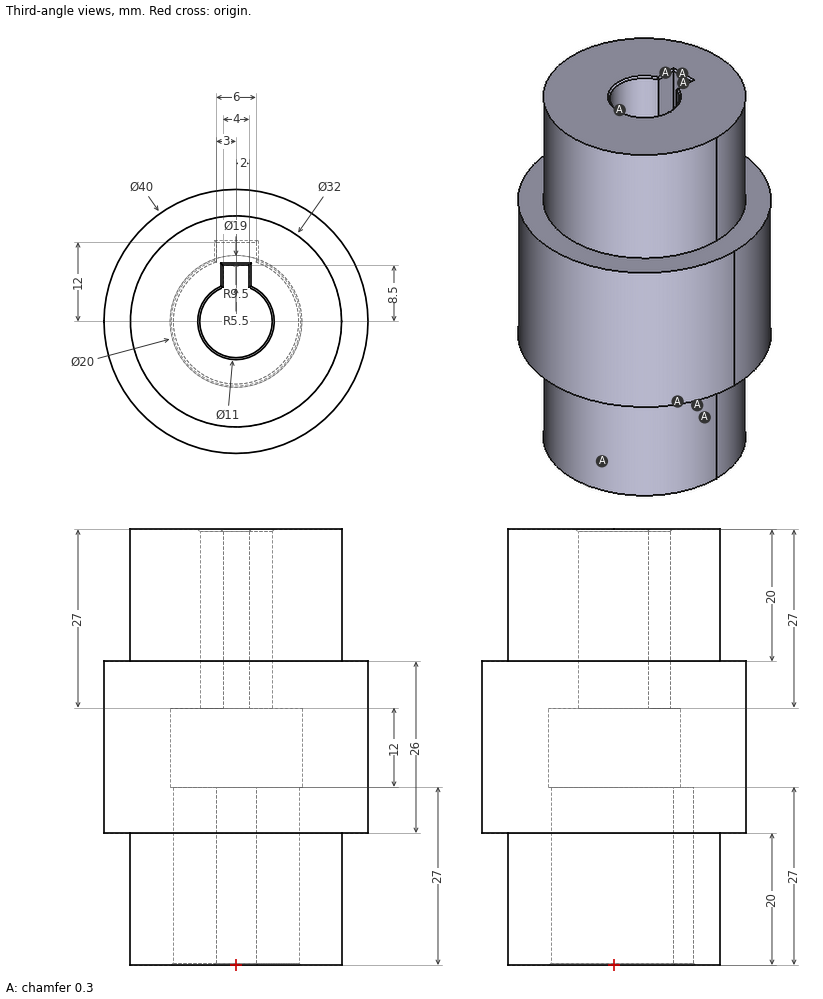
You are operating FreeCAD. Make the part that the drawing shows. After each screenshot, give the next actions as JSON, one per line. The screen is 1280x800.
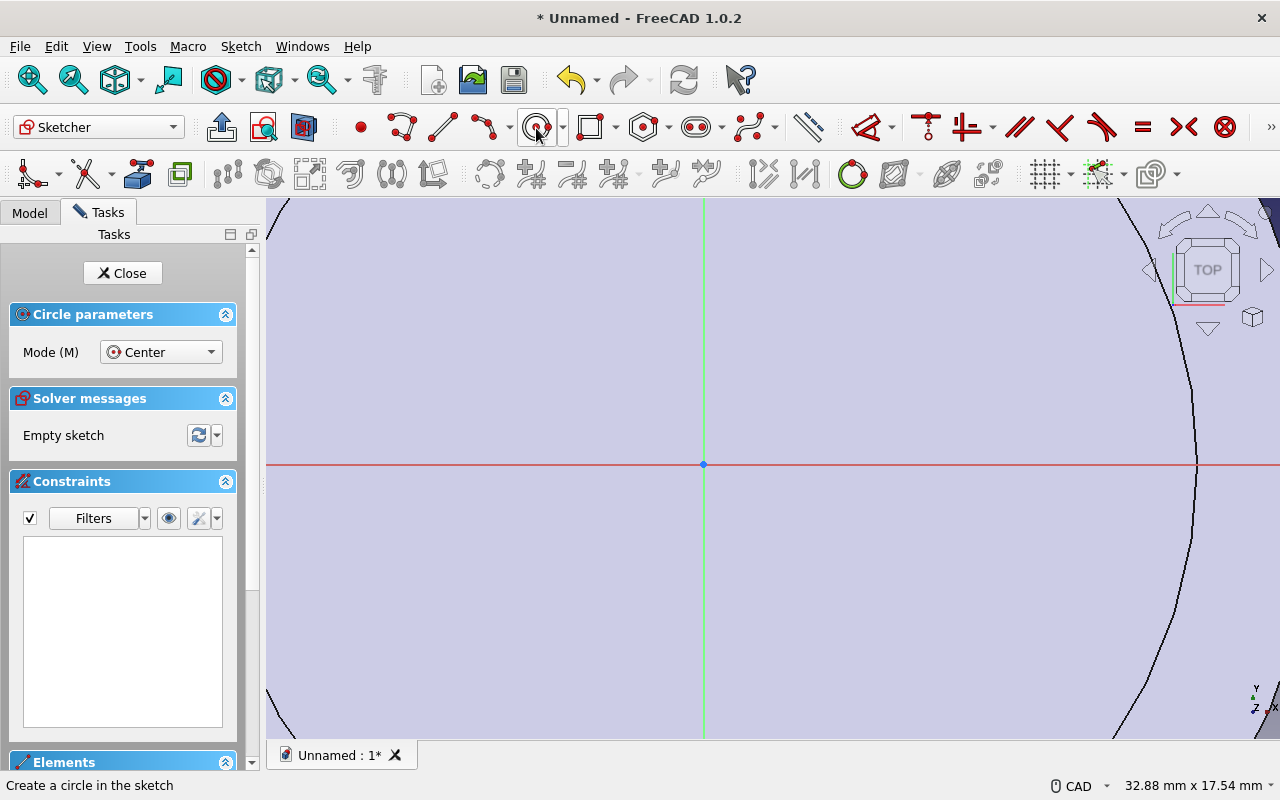
{"action": "left_click", "coordinate": [704, 465]}
{"action": "left_click", "coordinate": [824, 345]}
{"action": "key", "text": "Escape"}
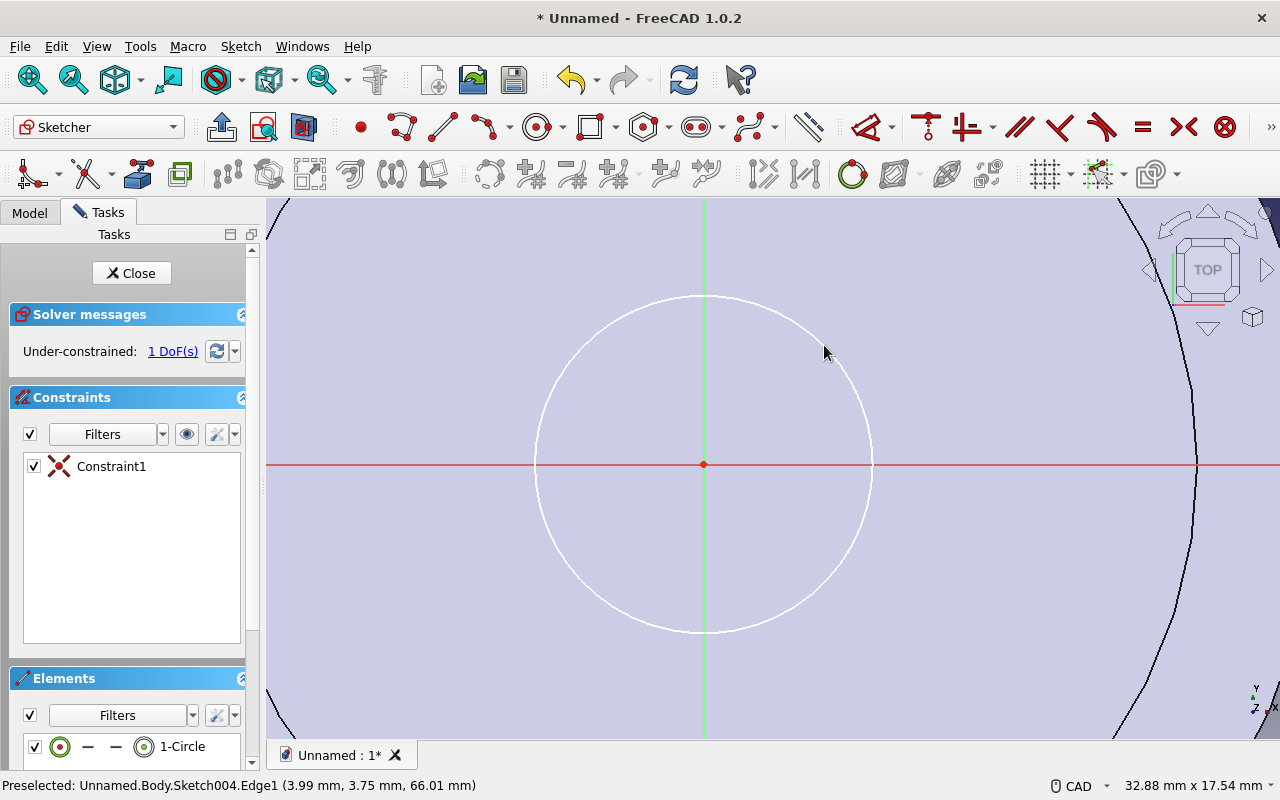
{"action": "left_click", "coordinate": [866, 128]}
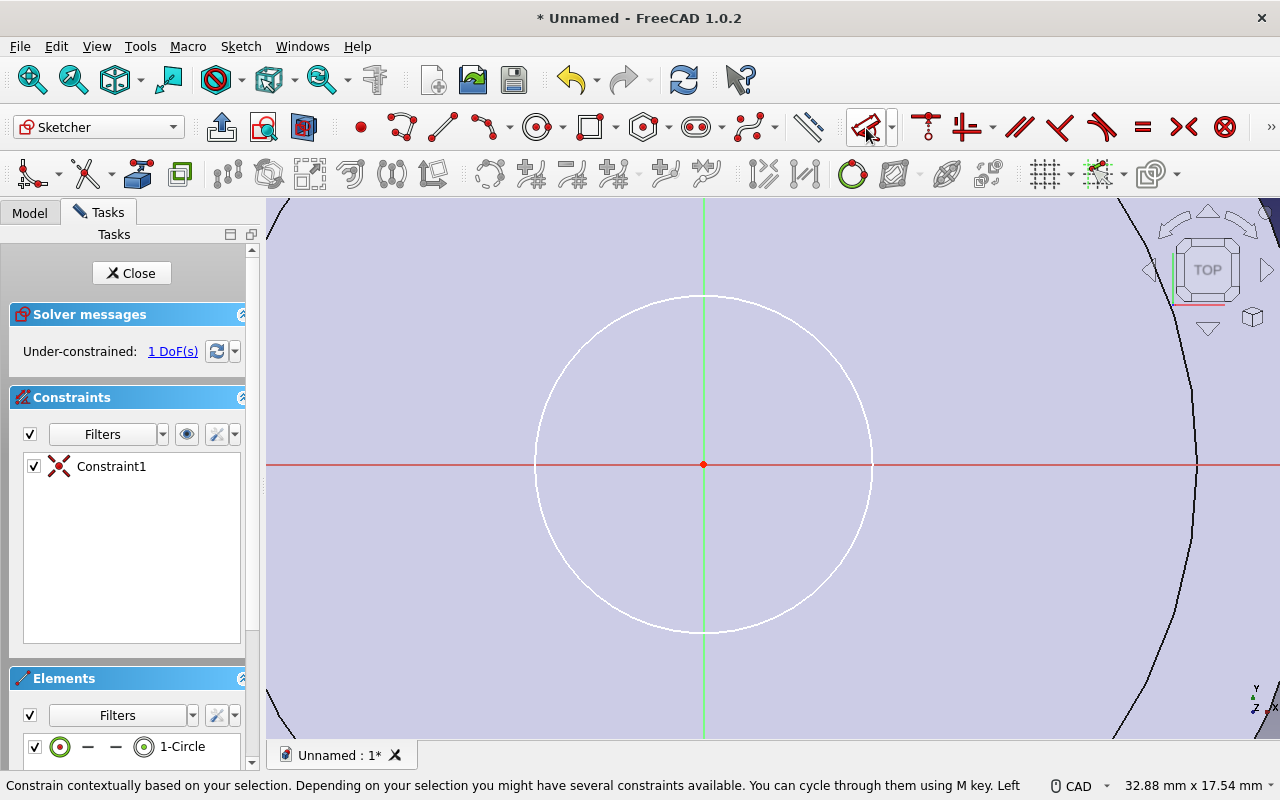
{"action": "left_click", "coordinate": [823, 345]}
{"action": "left_click", "coordinate": [846, 322]}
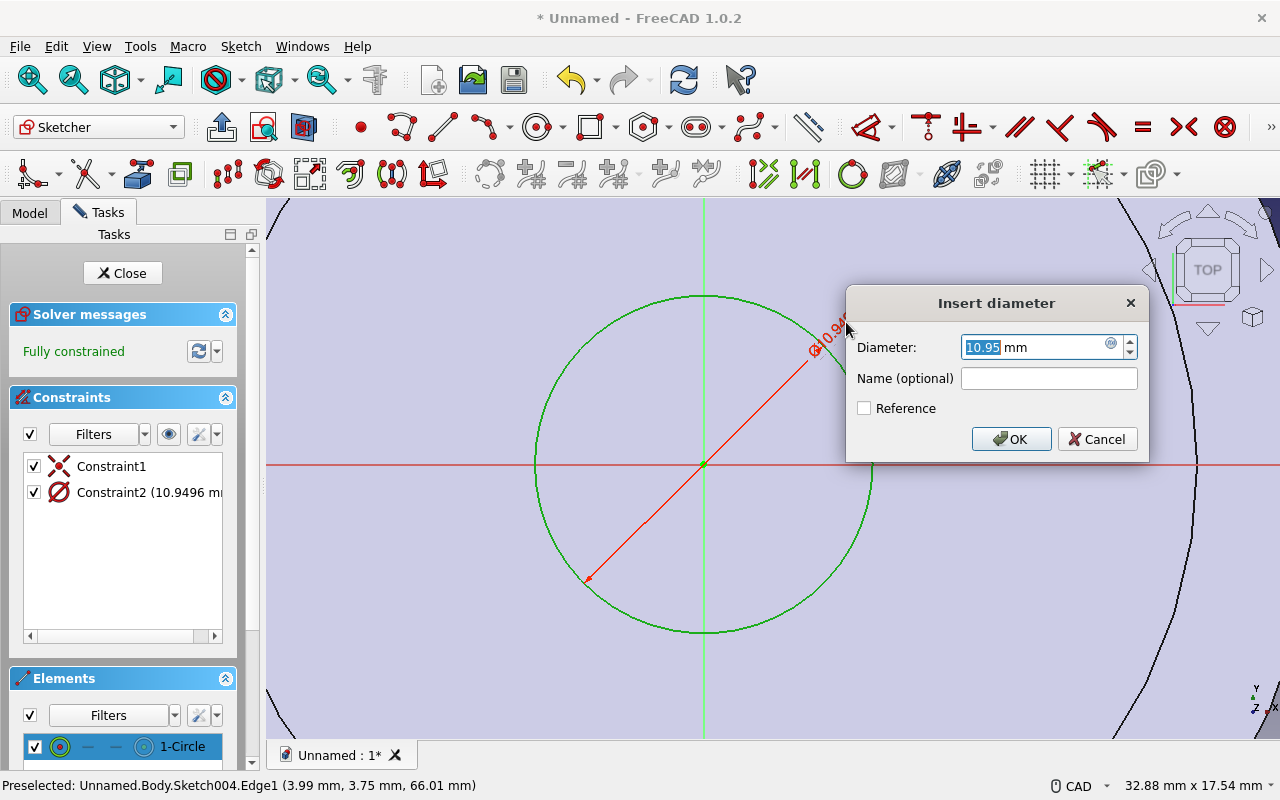
{"action": "type", "text": "11"}
{"action": "key", "text": "Return"}
{"action": "key", "text": "Escape"}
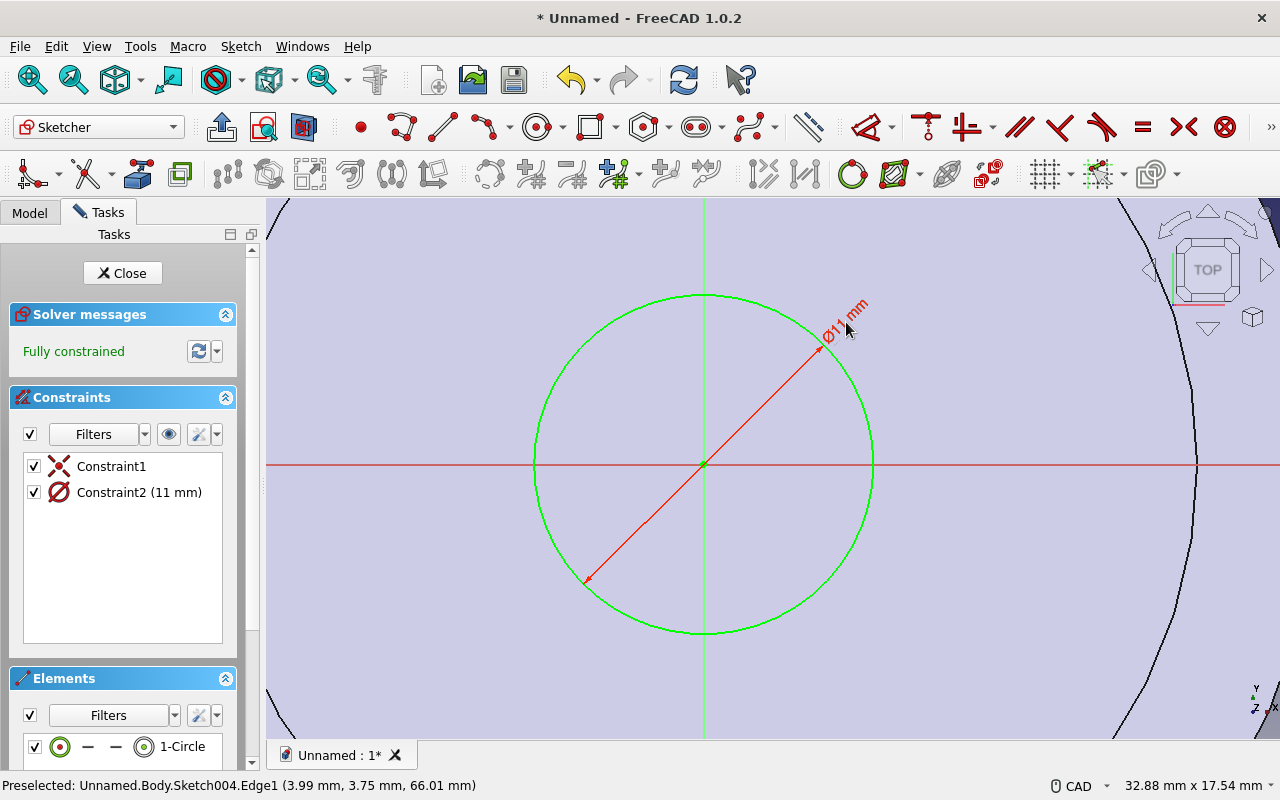
{"action": "left_click", "coordinate": [123, 273]}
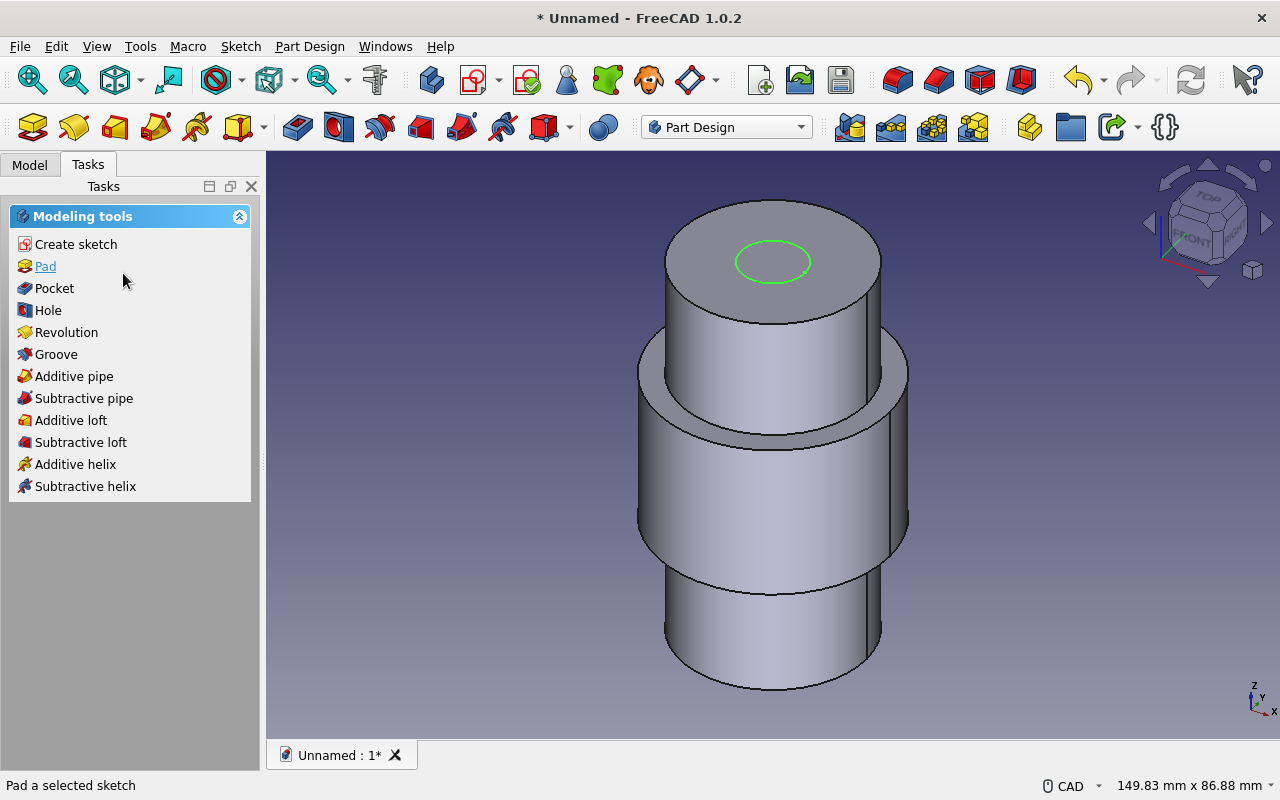
{"action": "left_click", "coordinate": [298, 128]}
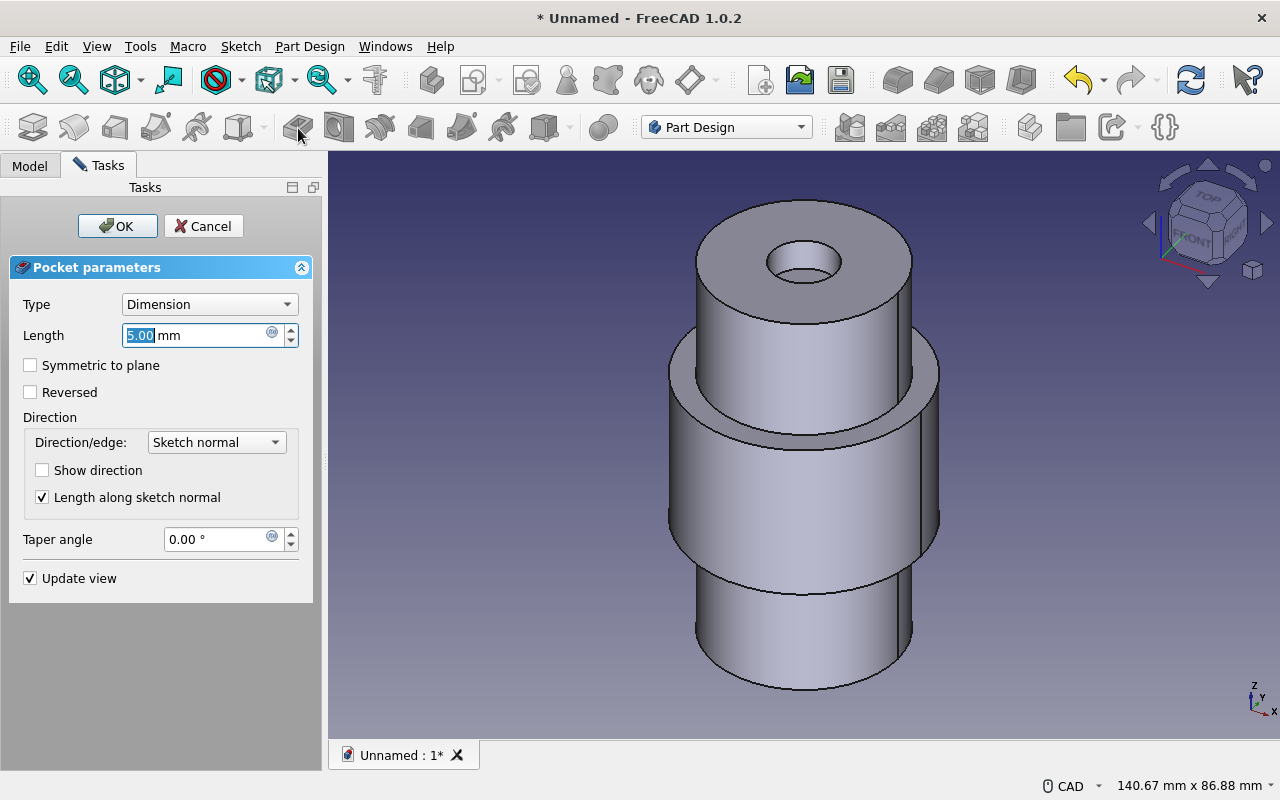
{"action": "type", "text": "27"}
{"action": "key", "text": "Tab"}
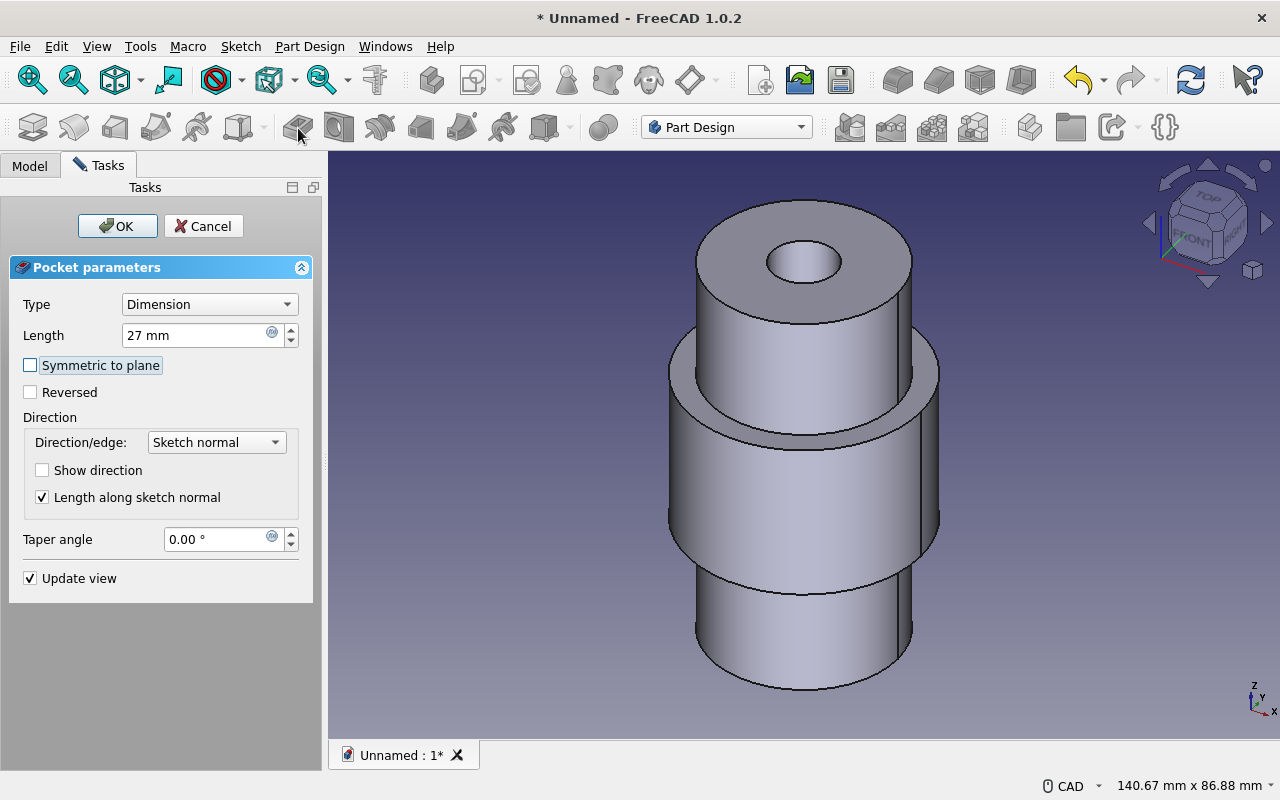
{"action": "left_click", "coordinate": [118, 226]}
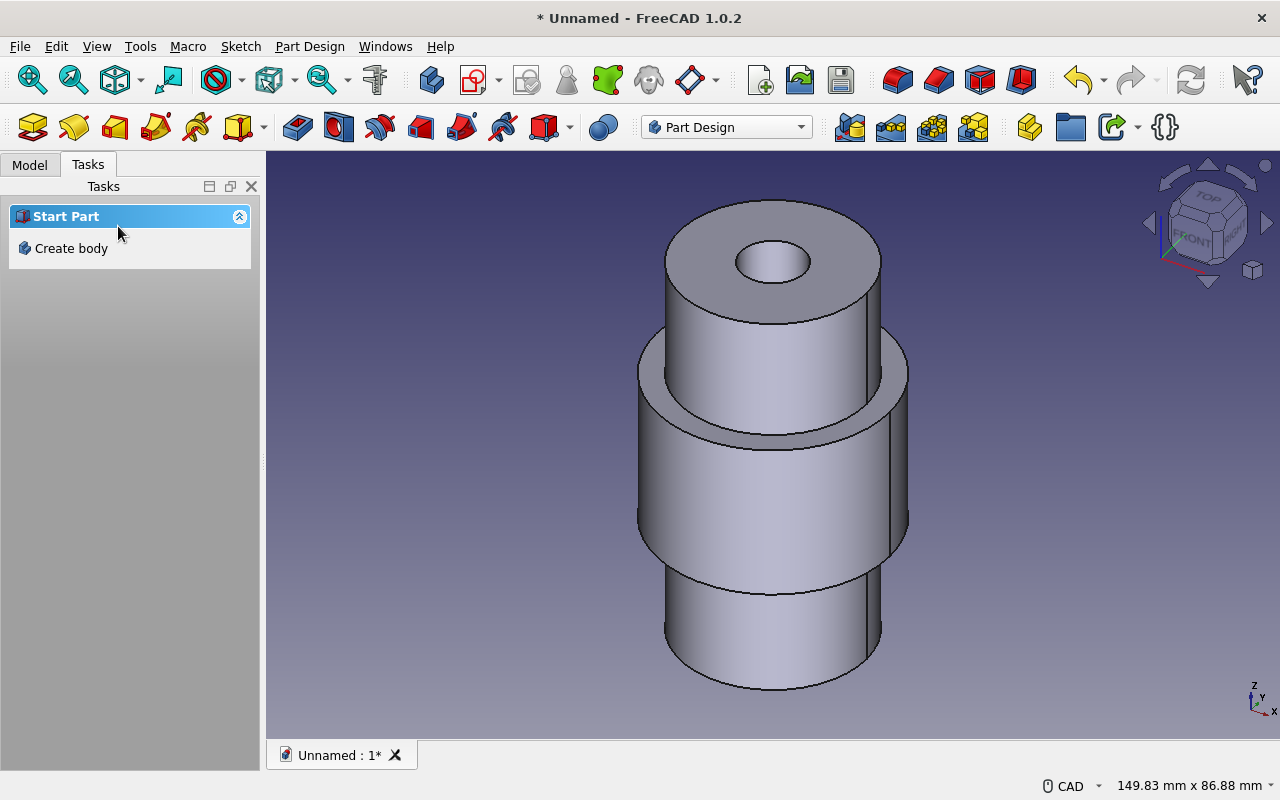
{"action": "key", "text": "0"}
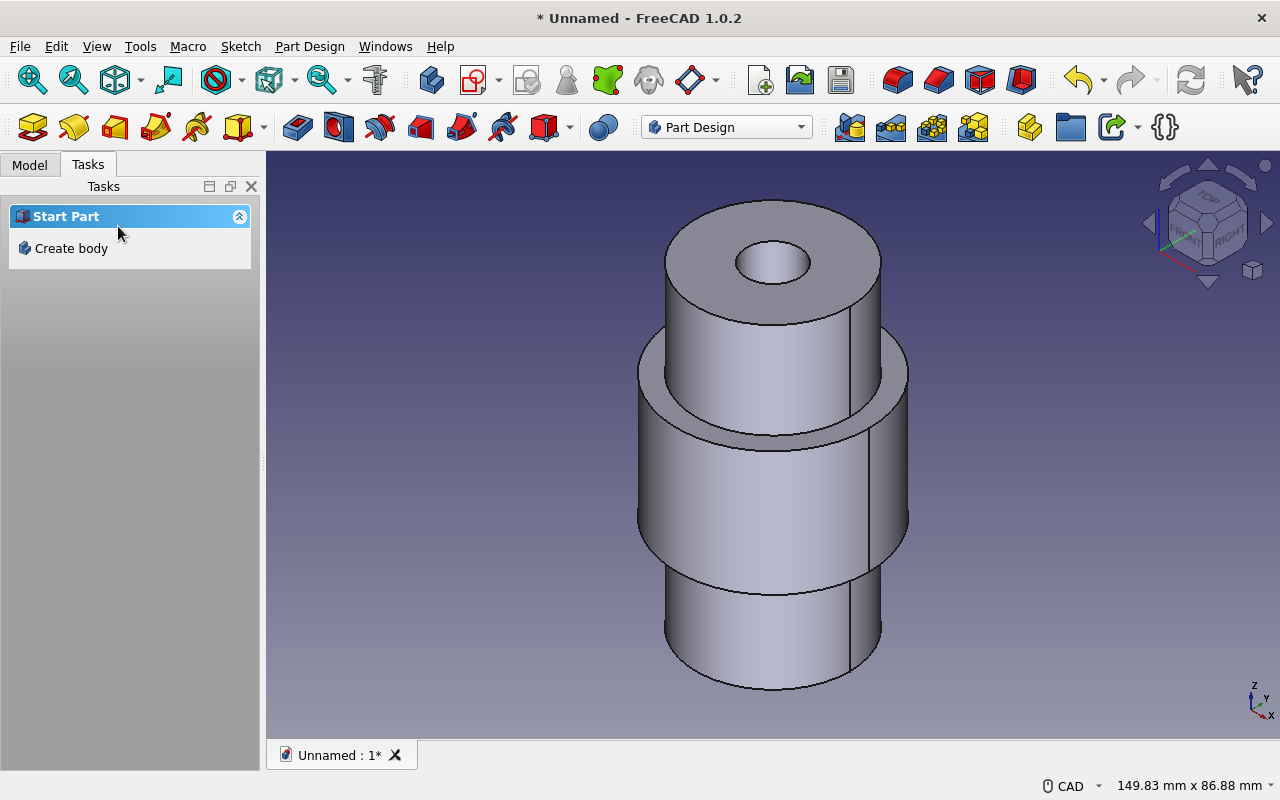
{"action": "key", "text": "2"}